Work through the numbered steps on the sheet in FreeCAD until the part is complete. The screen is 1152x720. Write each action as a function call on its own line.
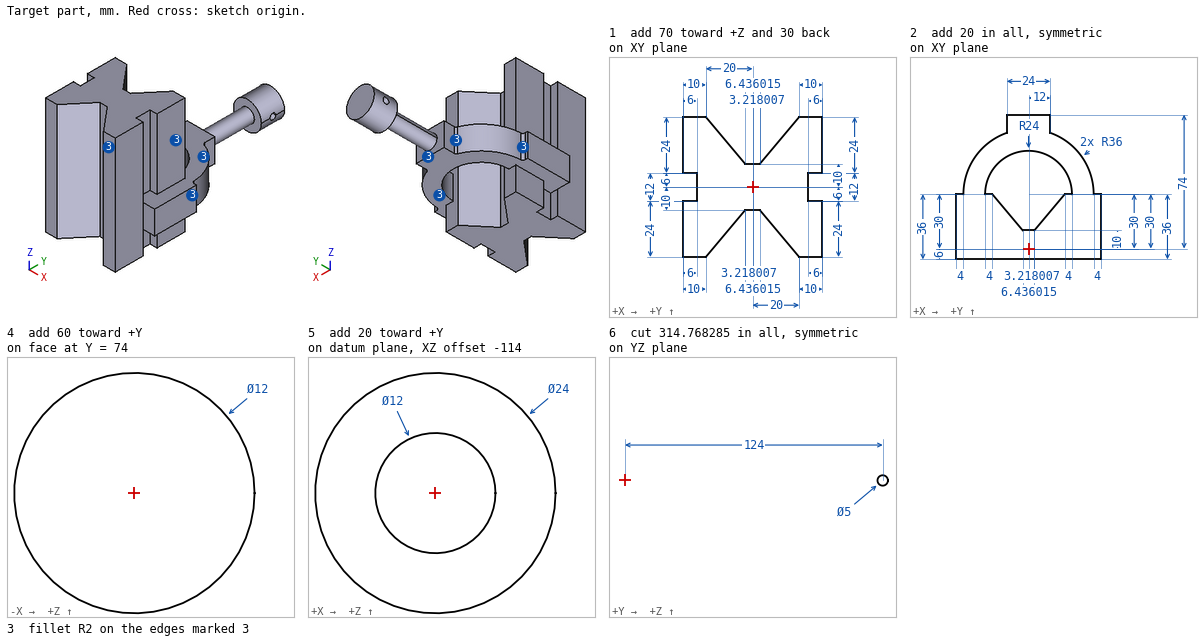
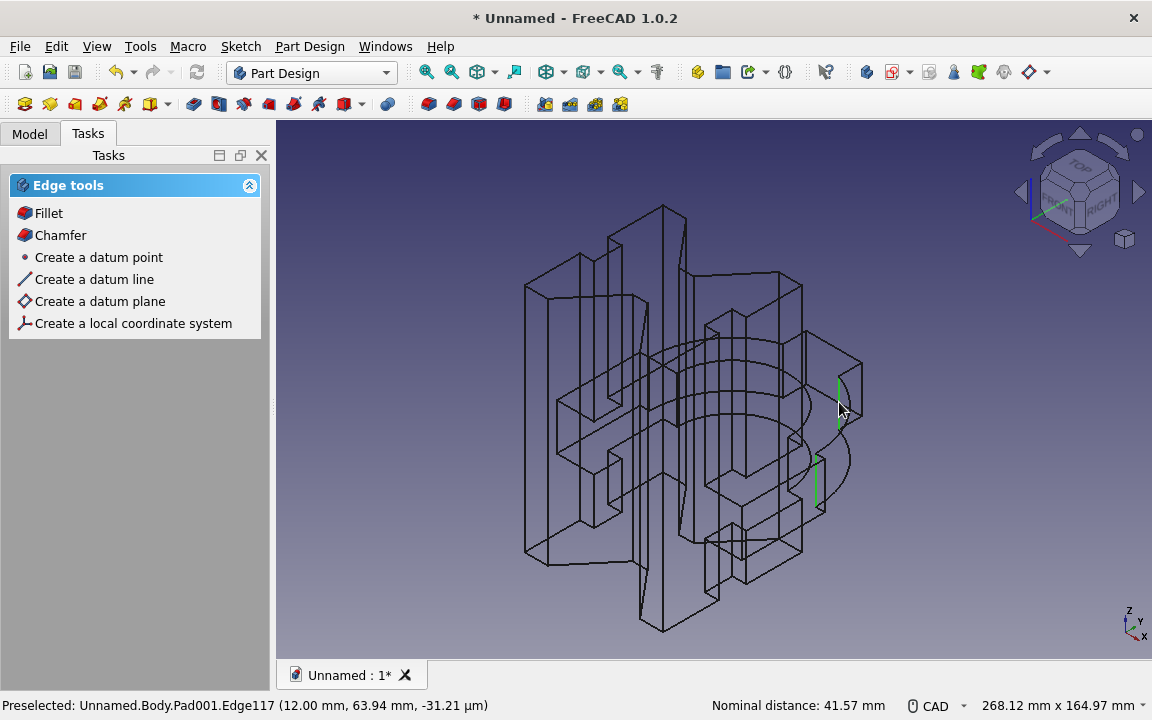
key(2)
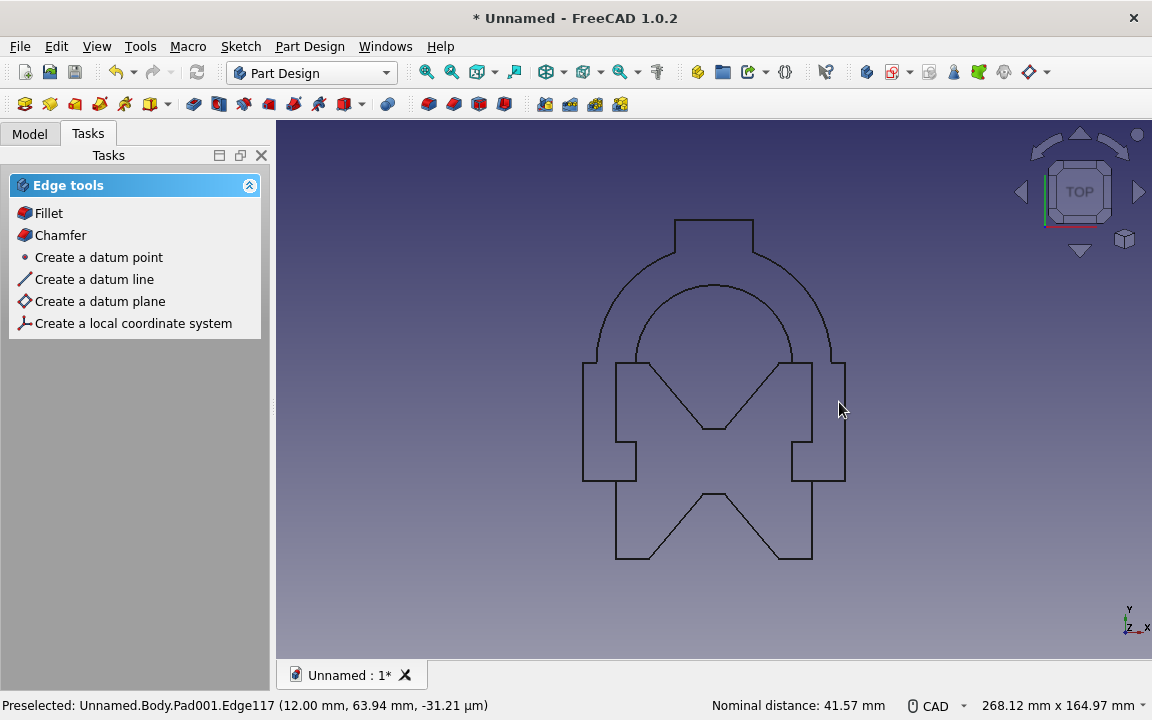
key(1)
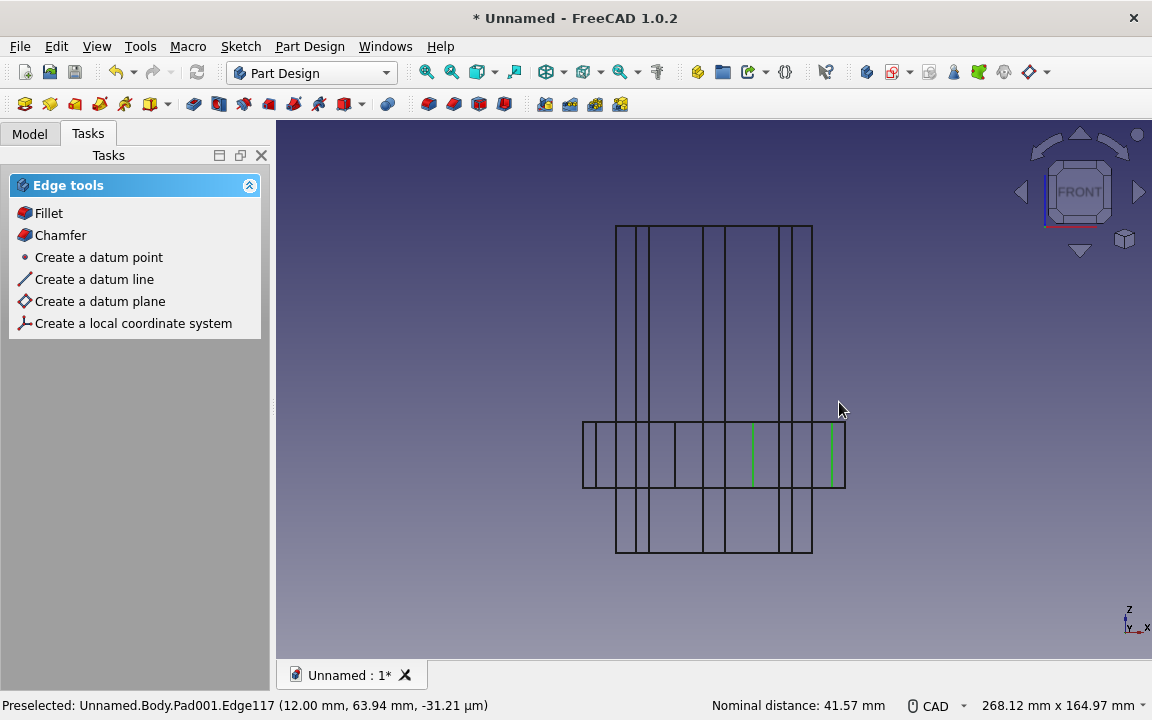
click(675, 454, ctrl)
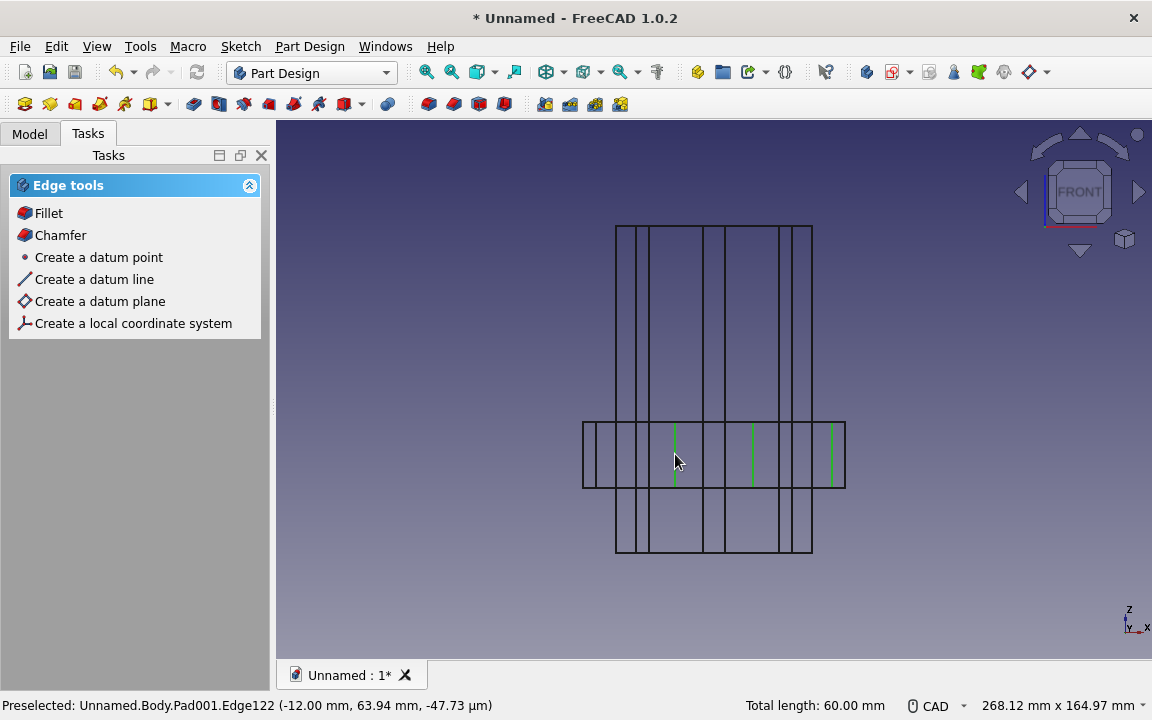
click(596, 454, ctrl)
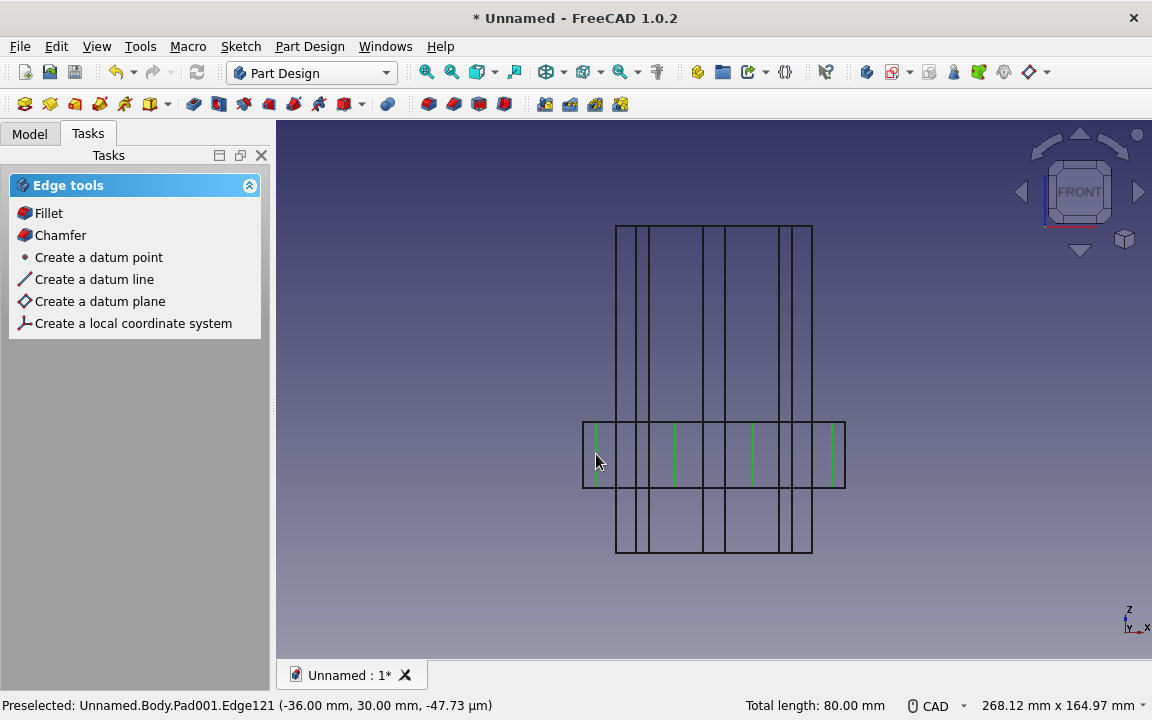
key(v)
key(1)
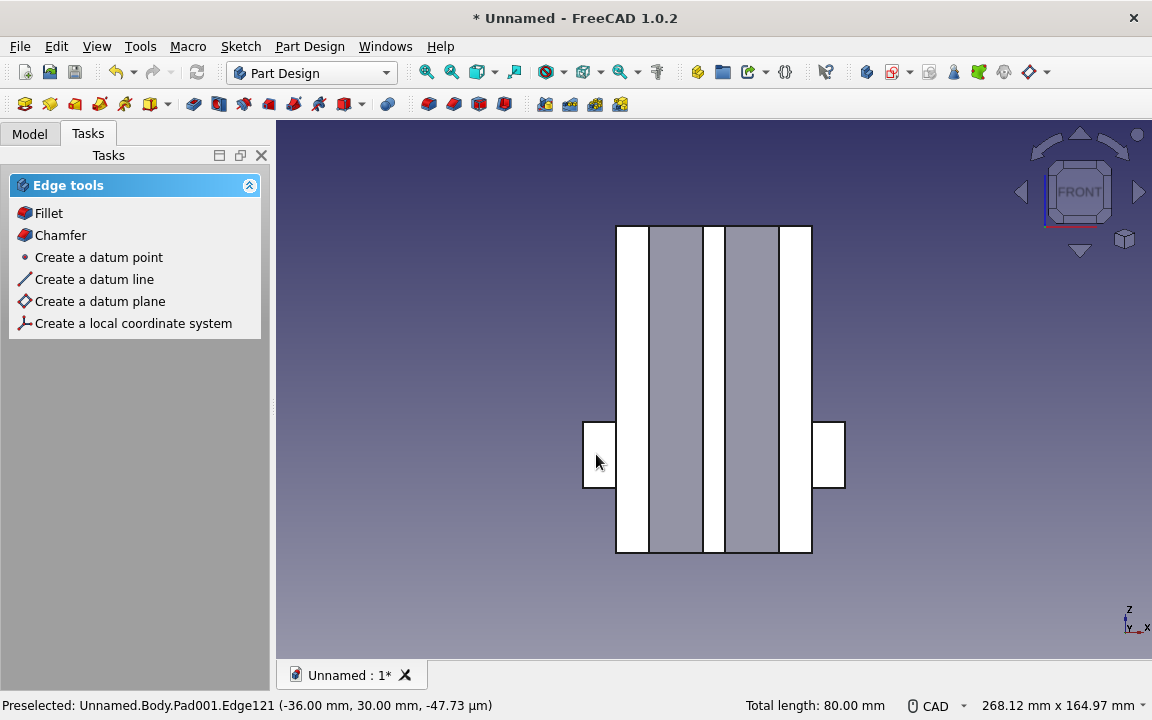
click(429, 104)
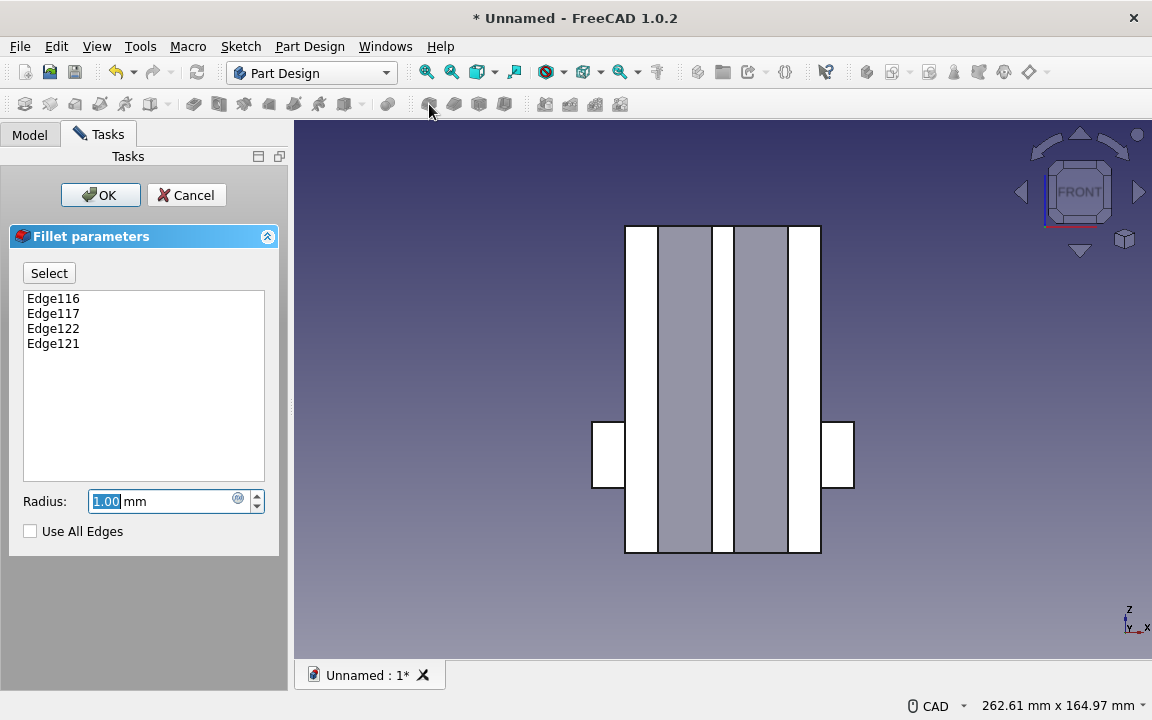
text(2)
key(Tab)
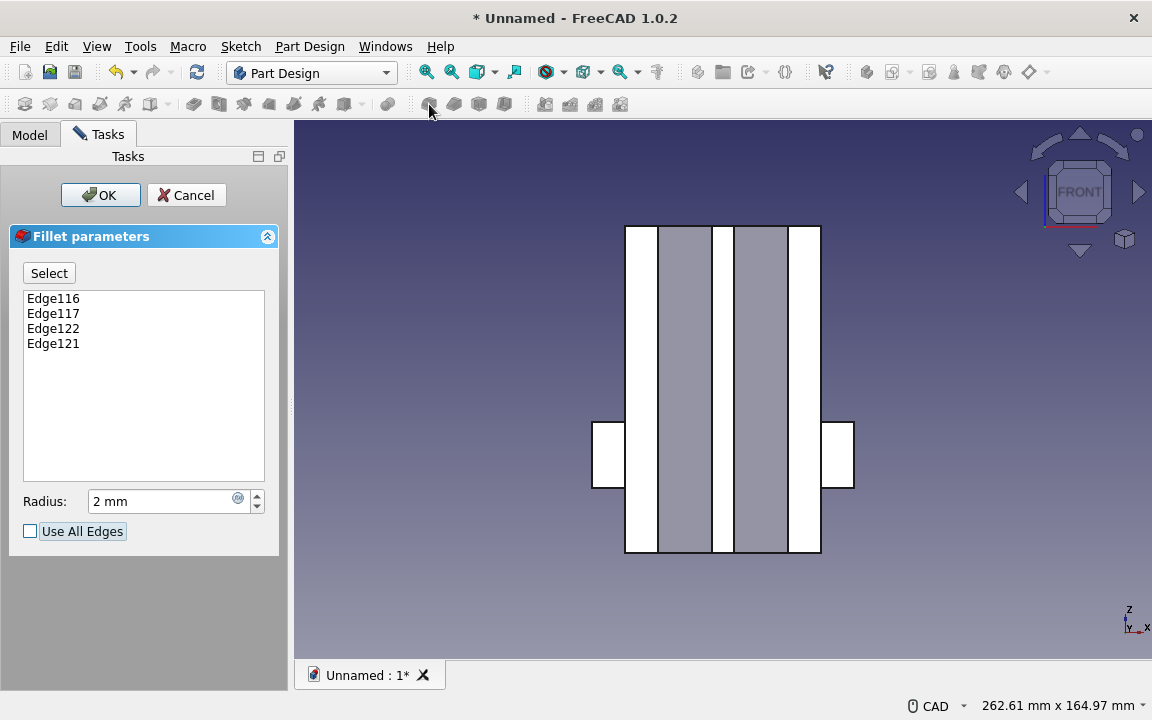
click(101, 195)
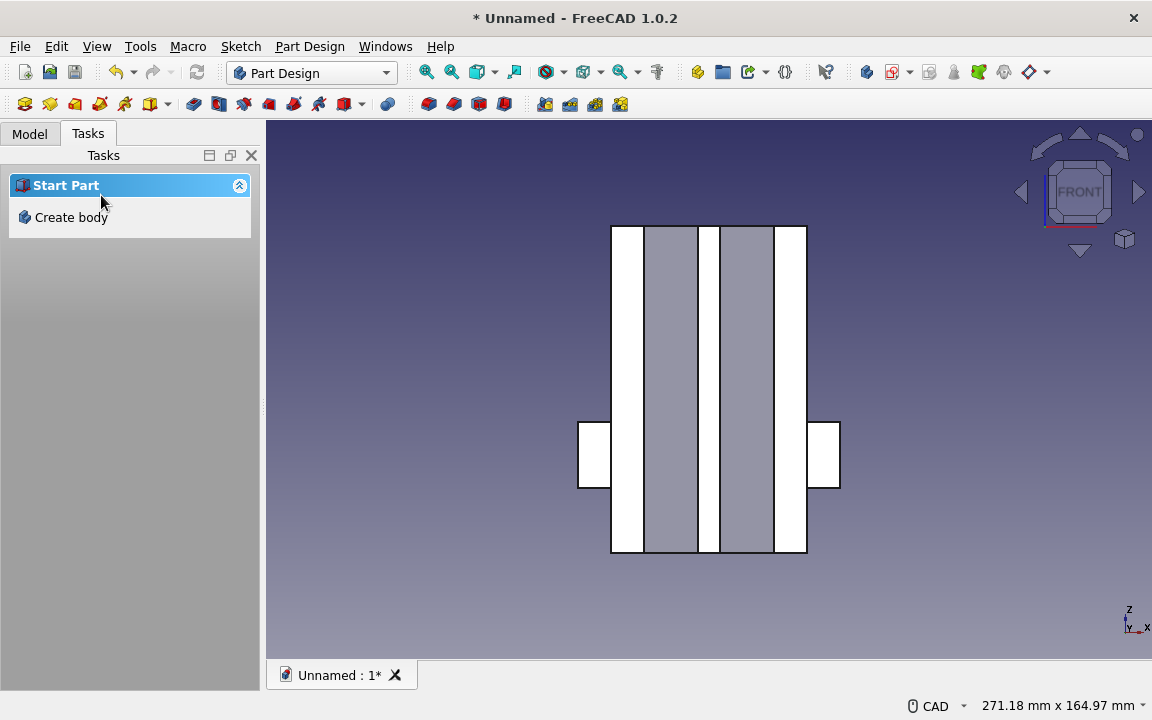
key(4)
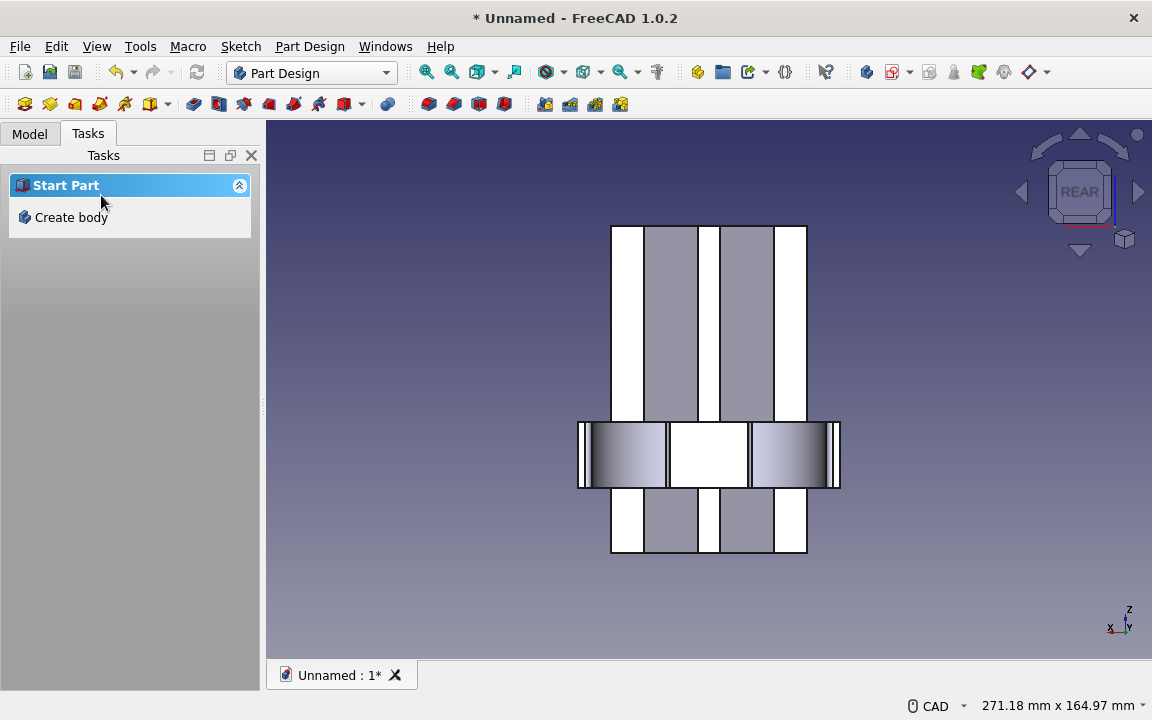
click(709, 454)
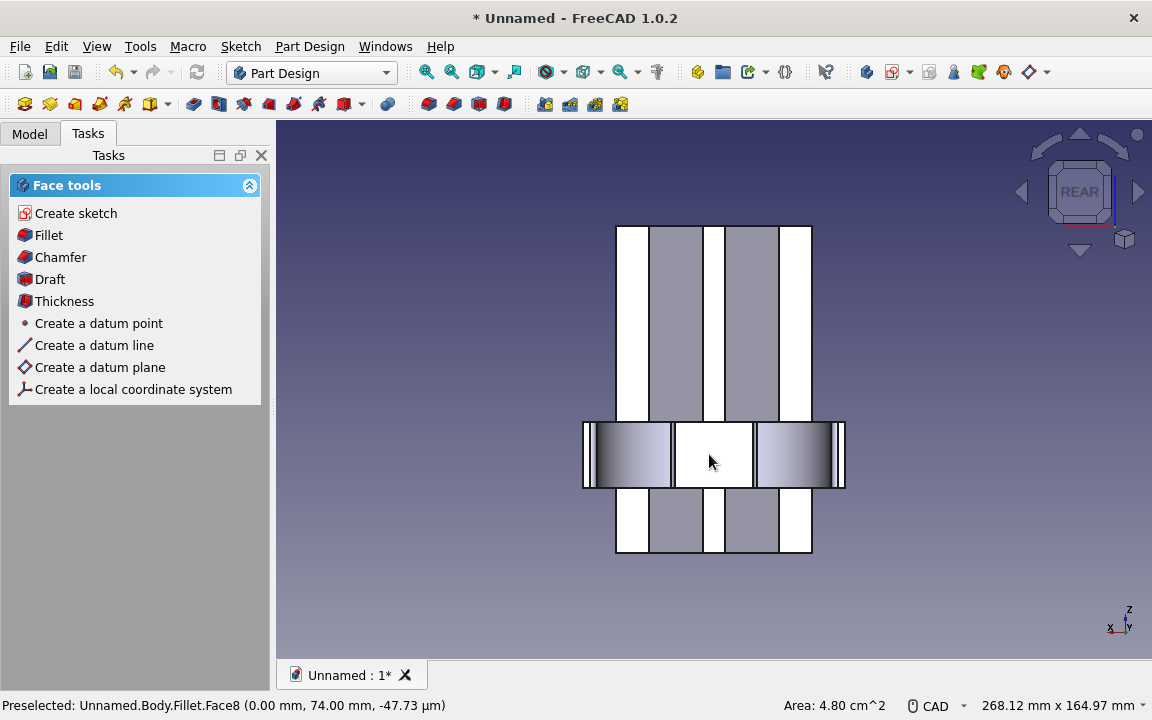
click(892, 72)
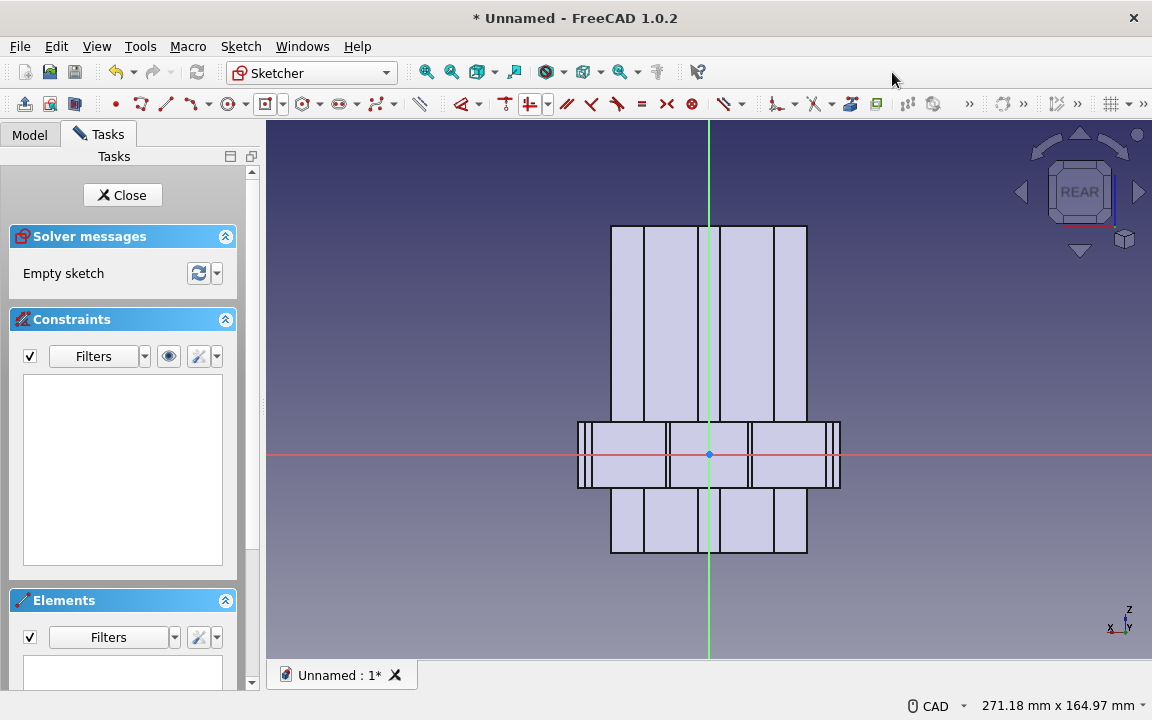
scroll(718, 463, up, 11)